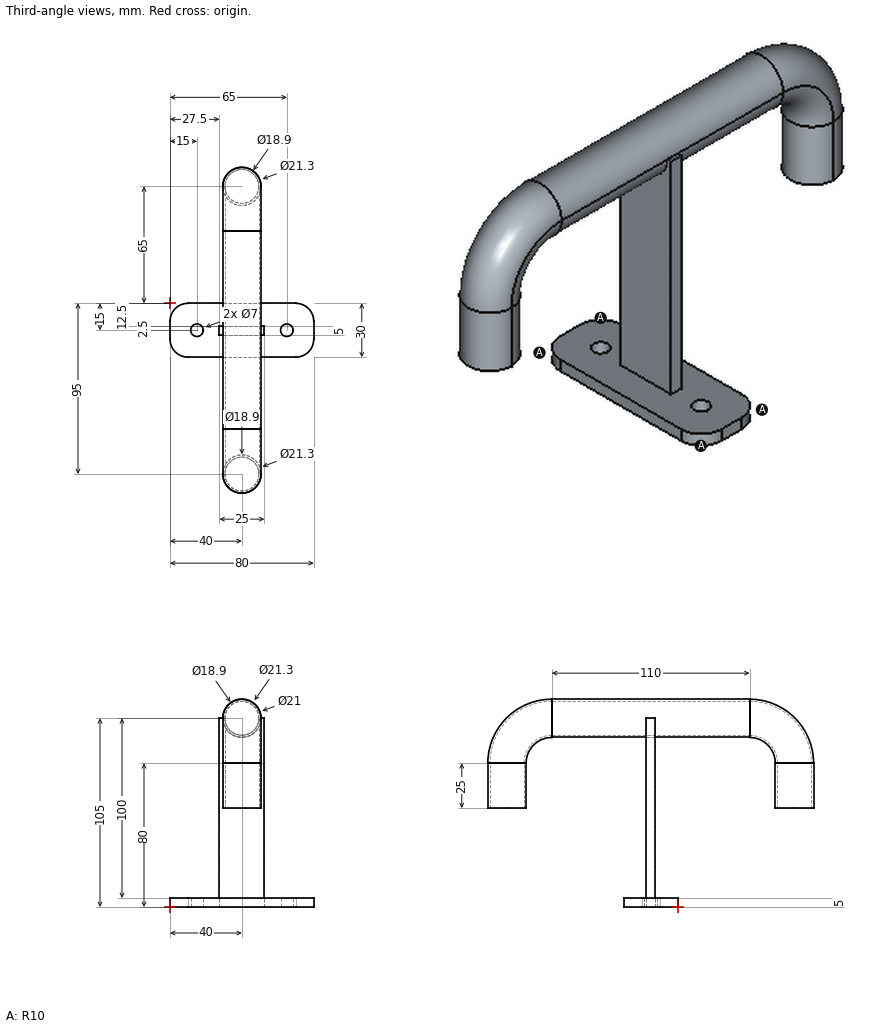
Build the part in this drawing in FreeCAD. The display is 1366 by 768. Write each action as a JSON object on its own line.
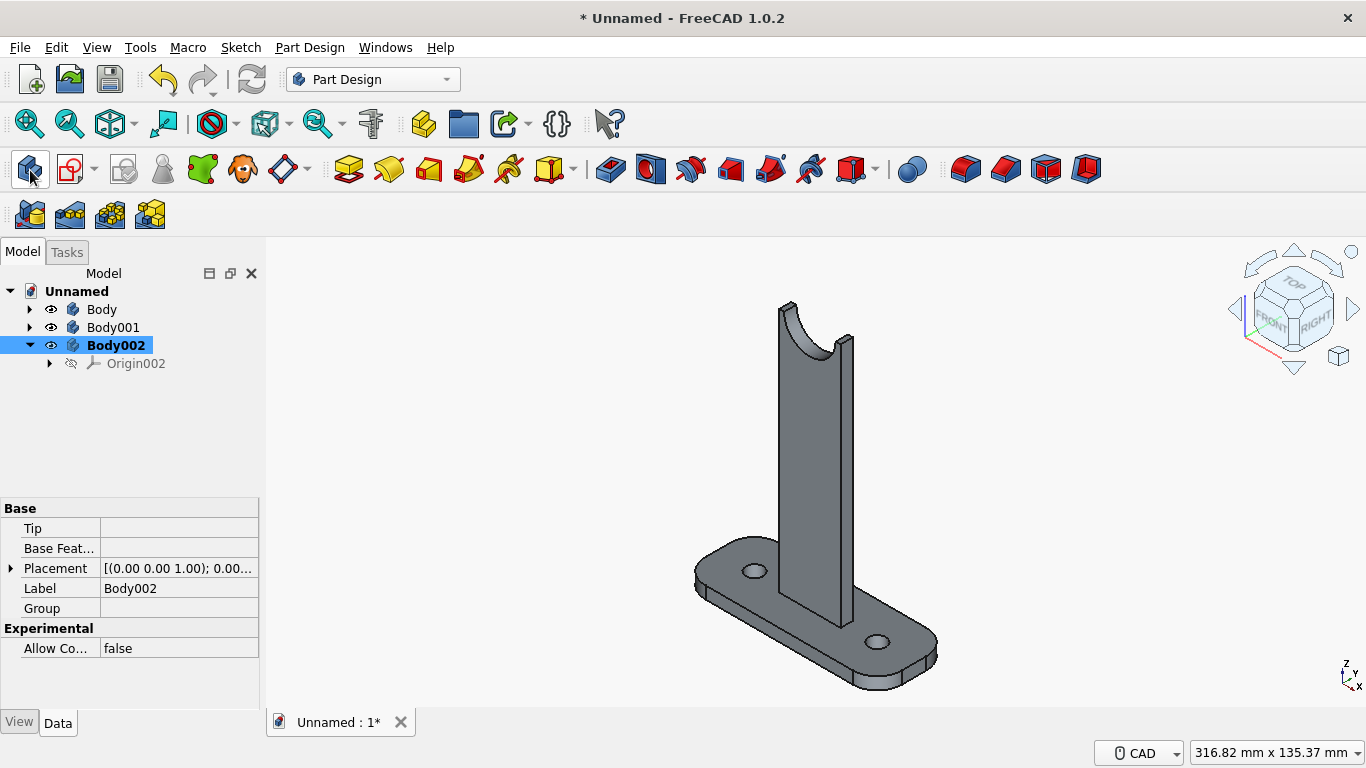
{"action": "left_click", "coordinate": [50, 363]}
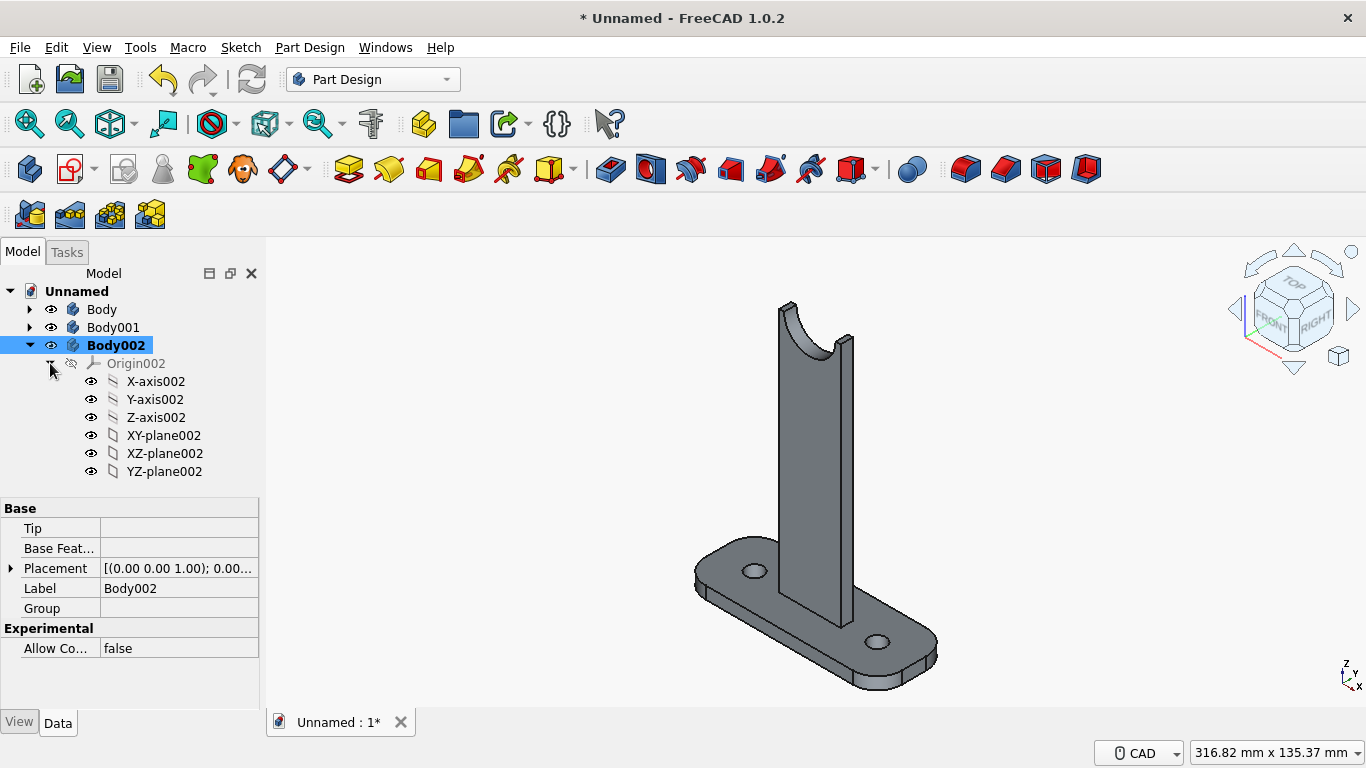
{"action": "left_click", "coordinate": [136, 453]}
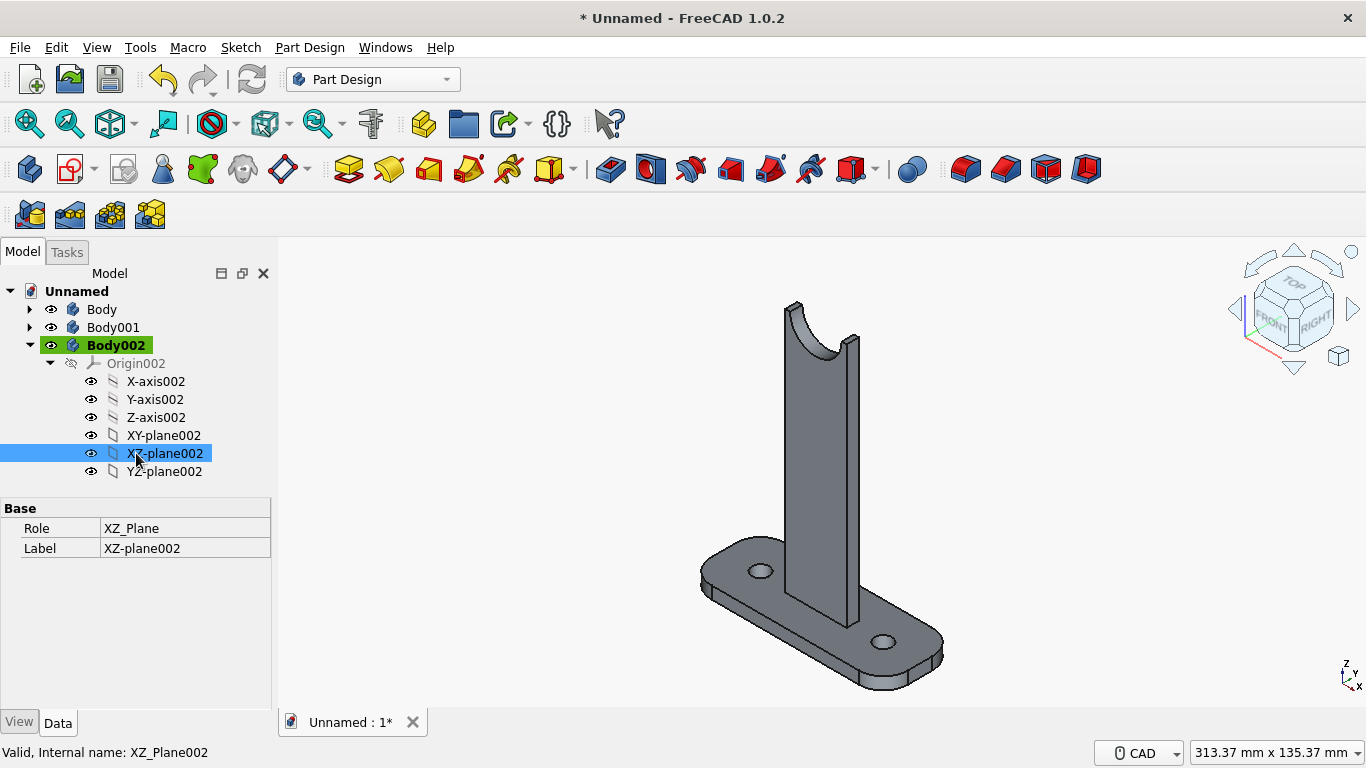
{"action": "left_click", "coordinate": [284, 170]}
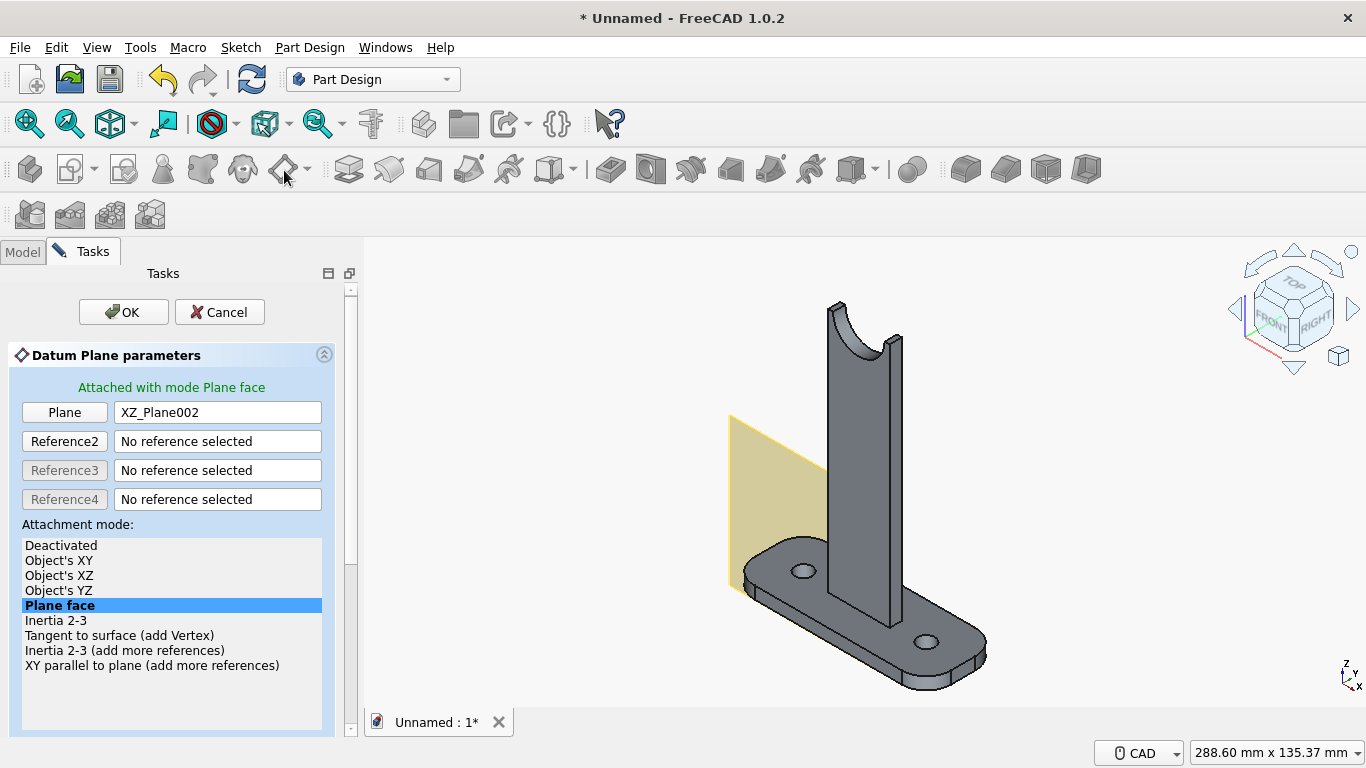
{"action": "scroll", "coordinate": [351, 510], "scroll_direction": "down", "scroll_amount": 3}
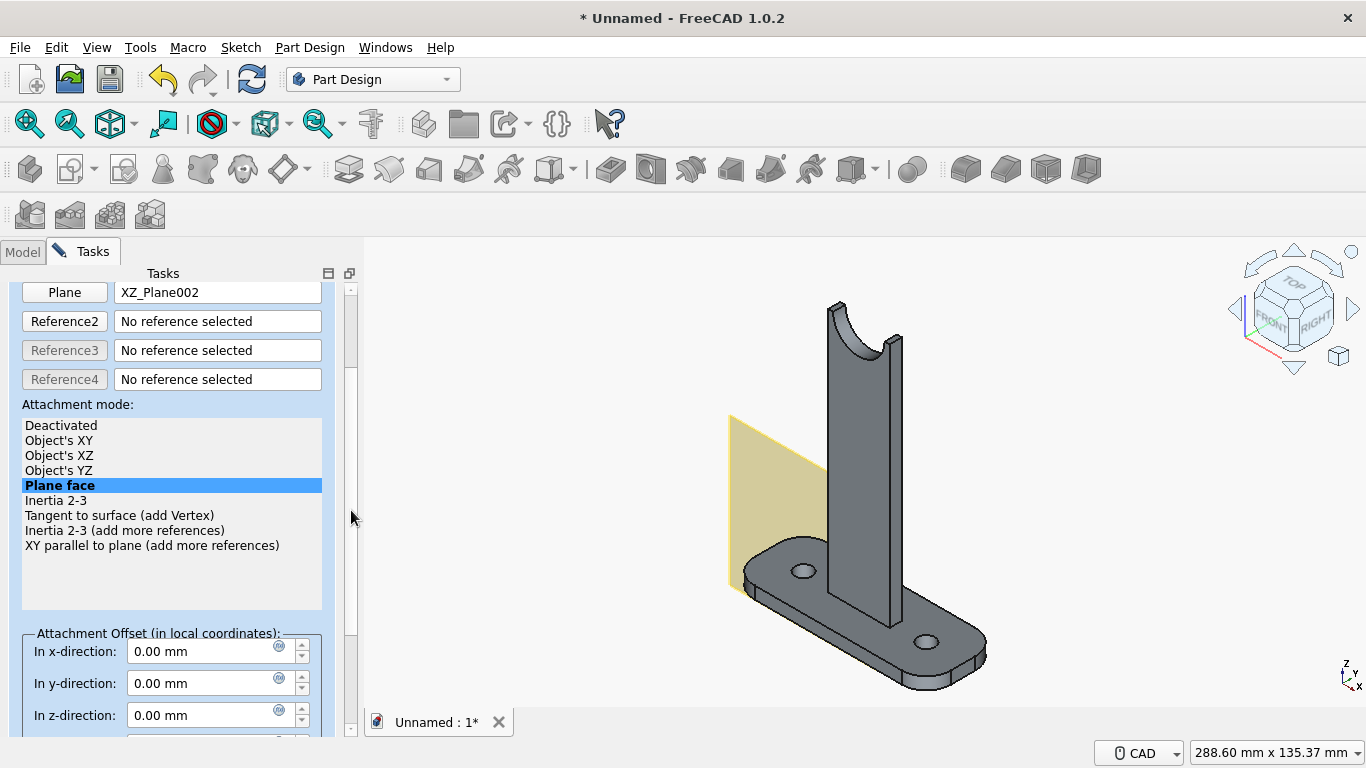
{"action": "triple_click", "coordinate": [210, 655]}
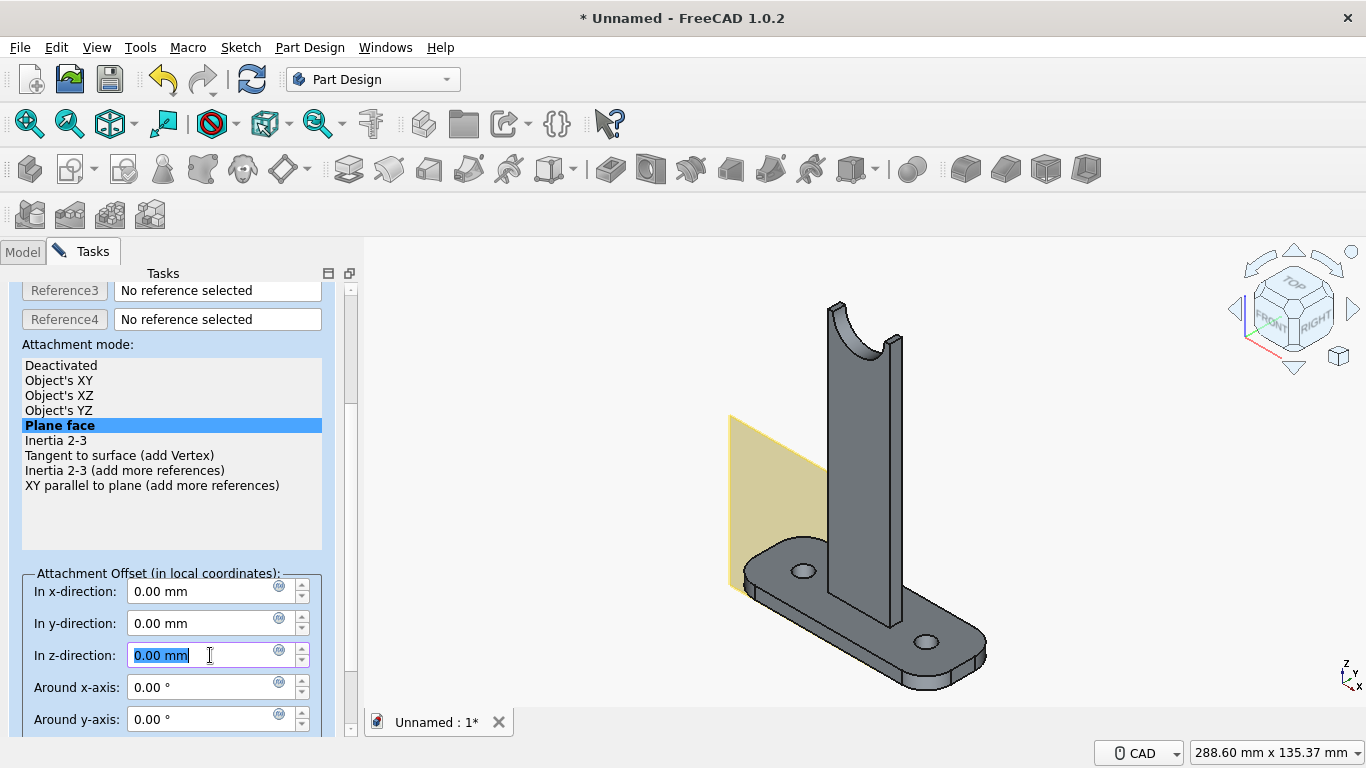
{"action": "type", "text": "-40"}
{"action": "key", "text": "Tab"}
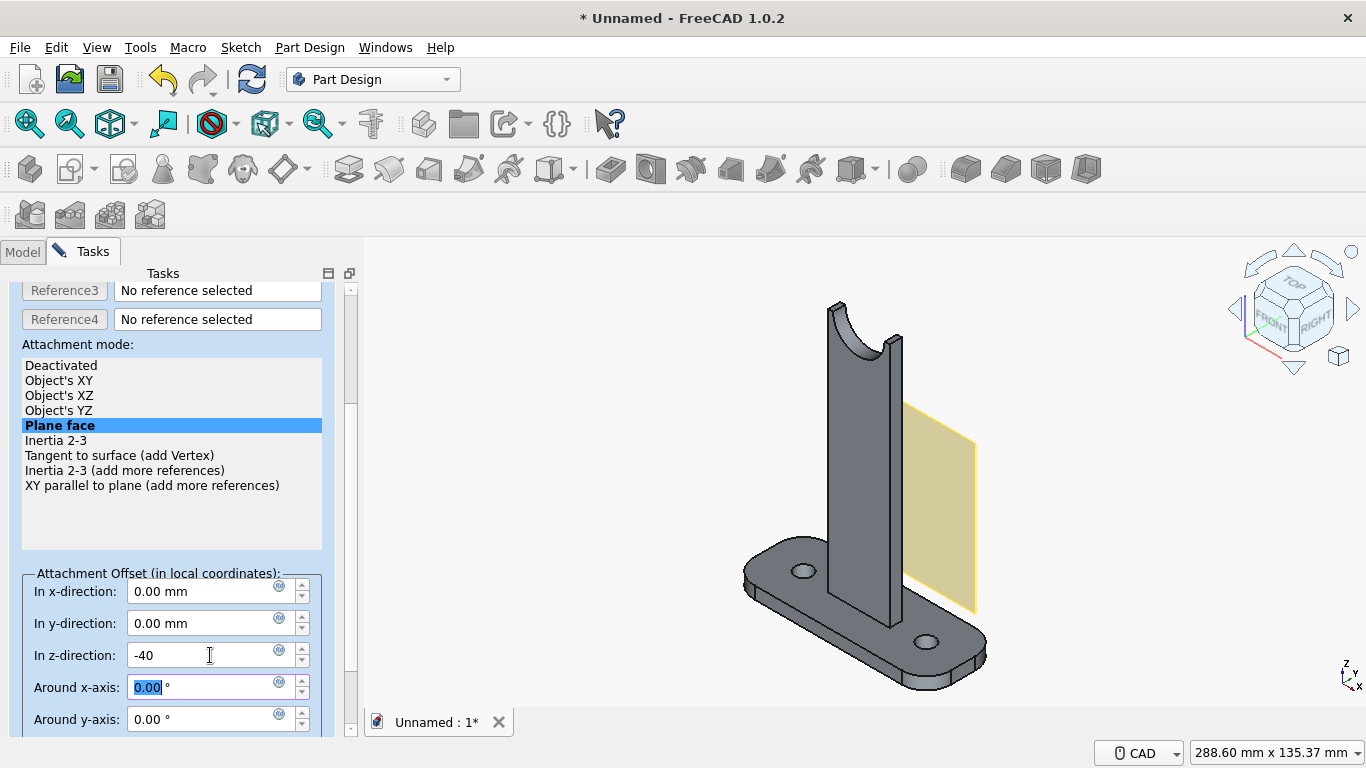
{"action": "scroll", "coordinate": [351, 510], "scroll_direction": "up", "scroll_amount": 4}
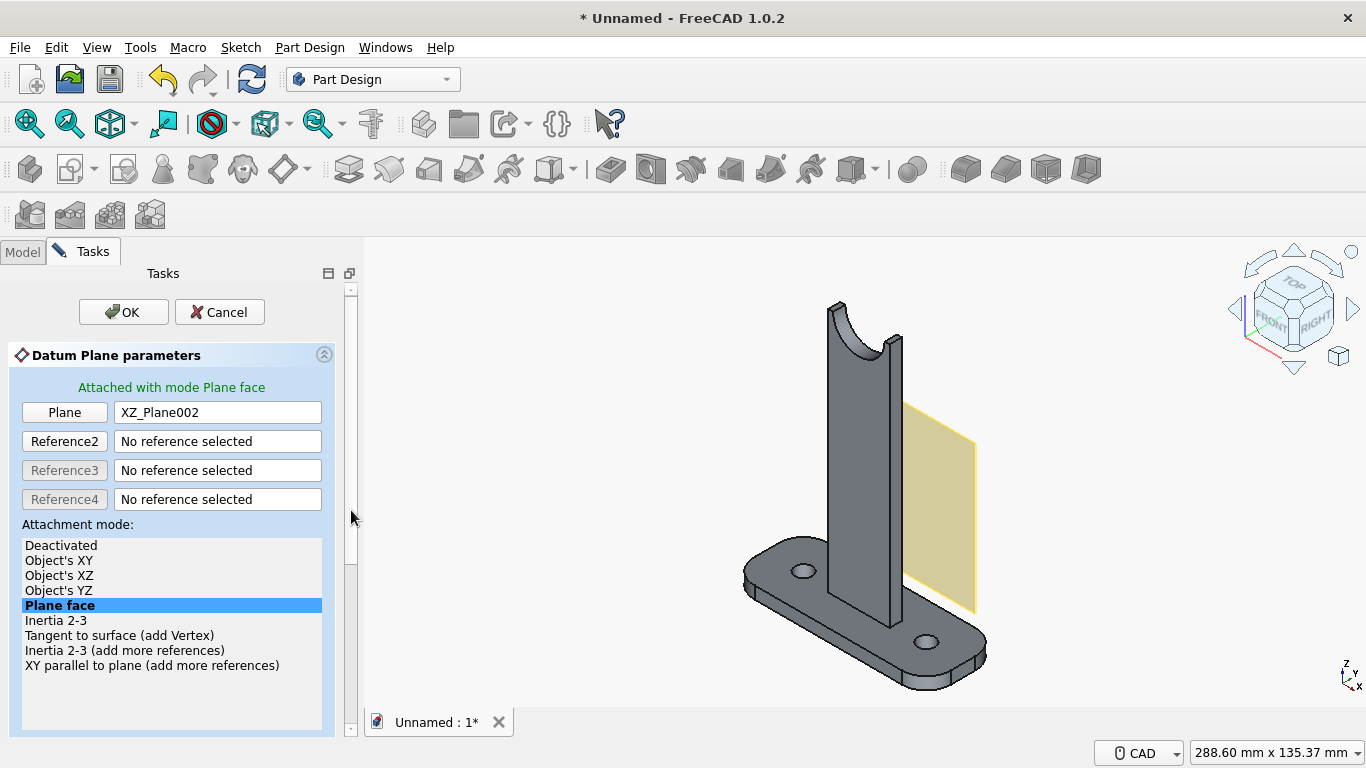
{"action": "left_click", "coordinate": [124, 312]}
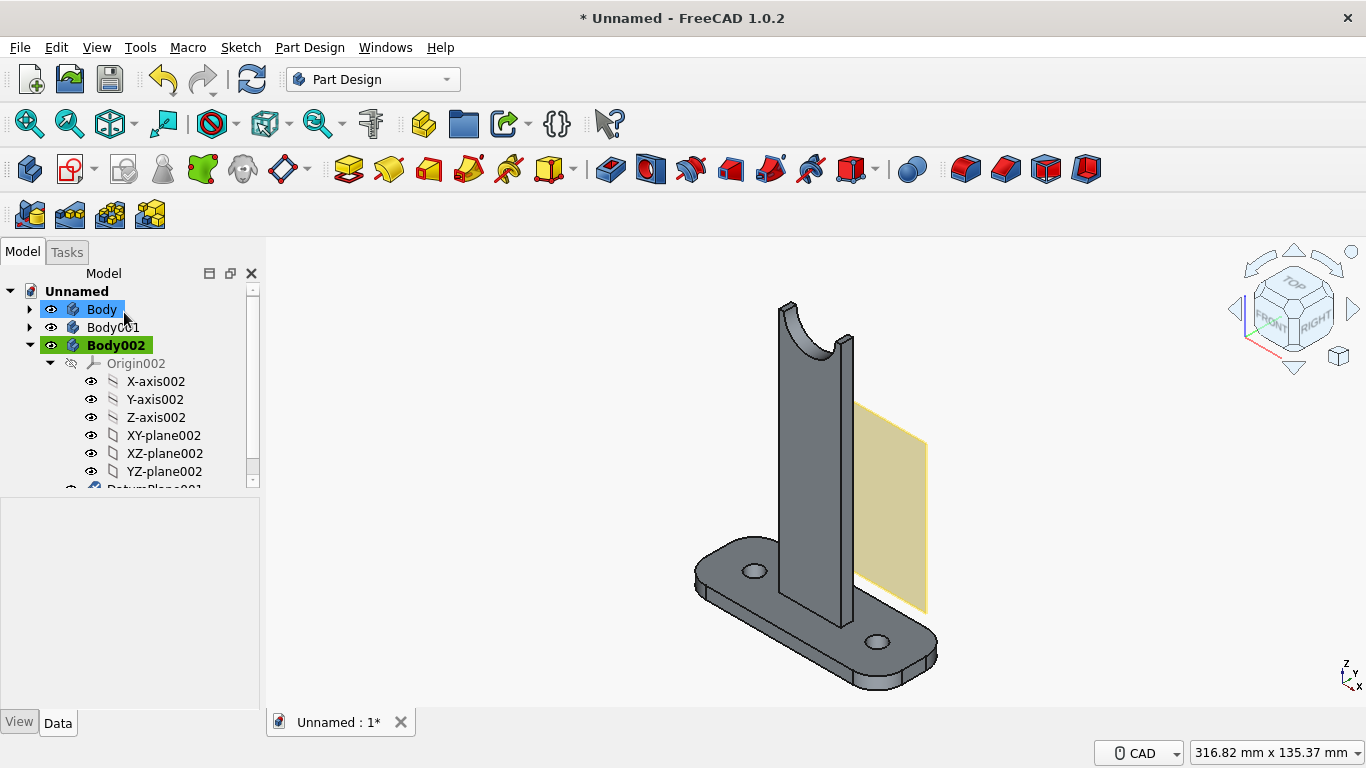
{"action": "scroll", "coordinate": [100, 377], "scroll_direction": "down", "scroll_amount": 3}